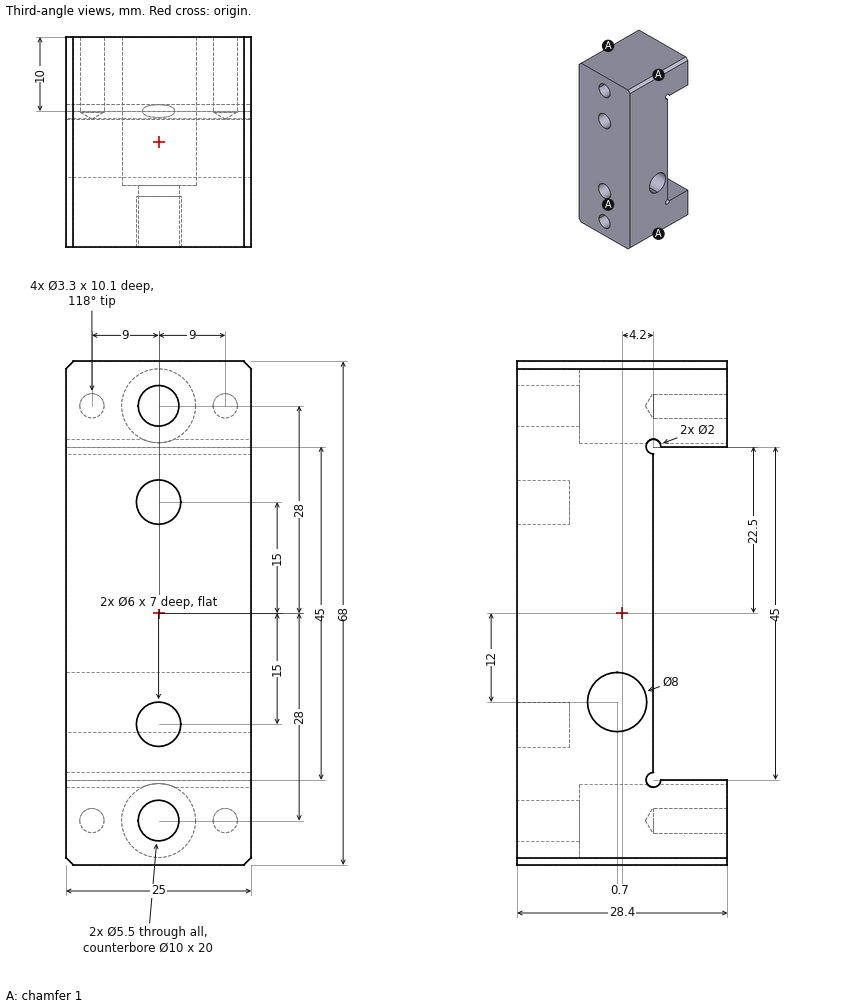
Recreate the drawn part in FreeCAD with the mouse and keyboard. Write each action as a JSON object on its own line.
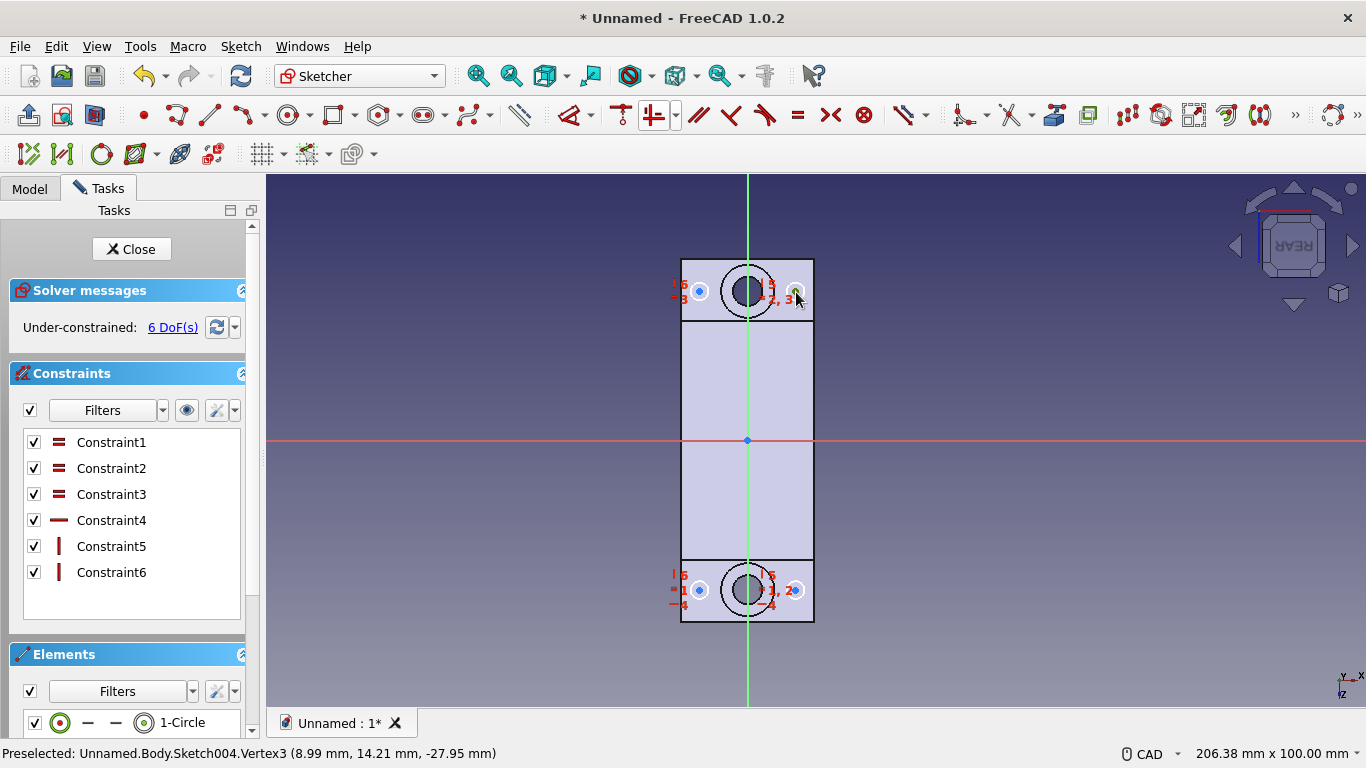
{"action": "left_click", "coordinate": [700, 292]}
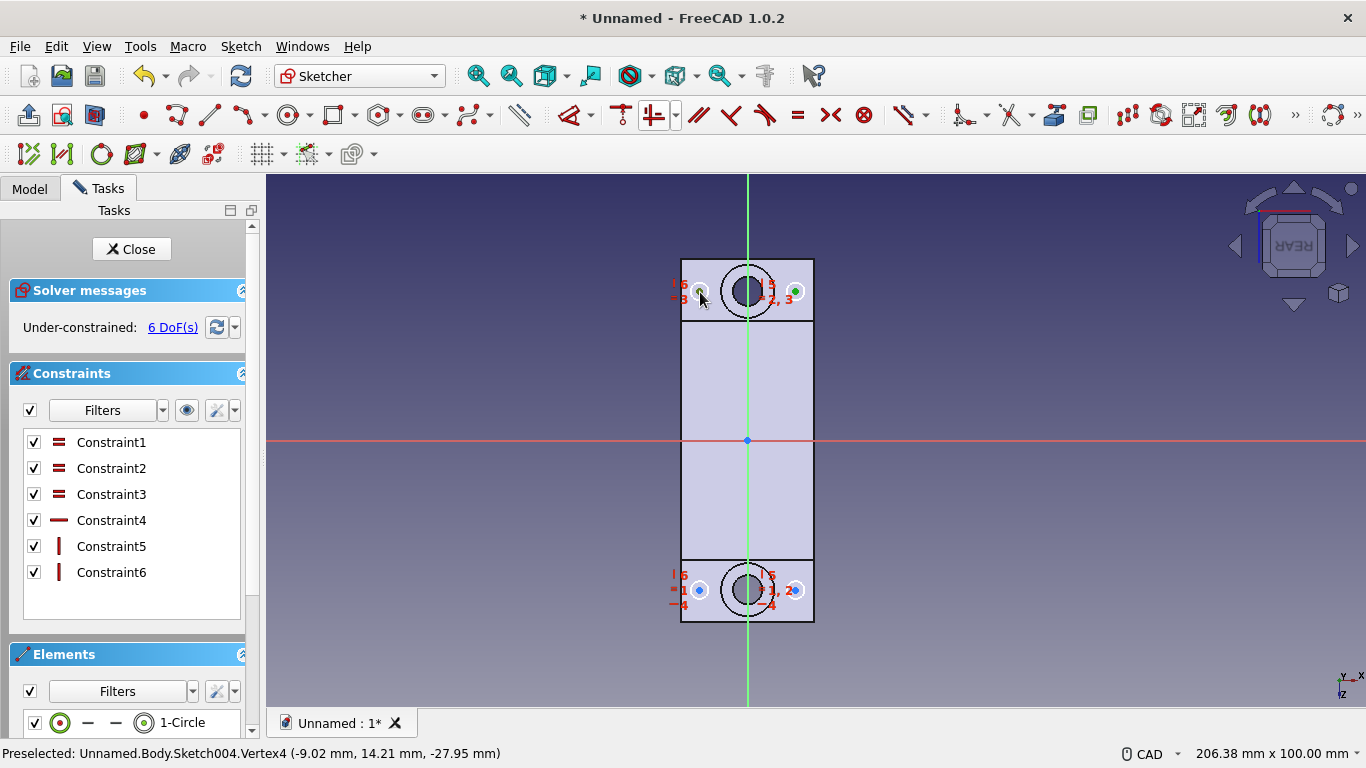
{"action": "key", "text": "h"}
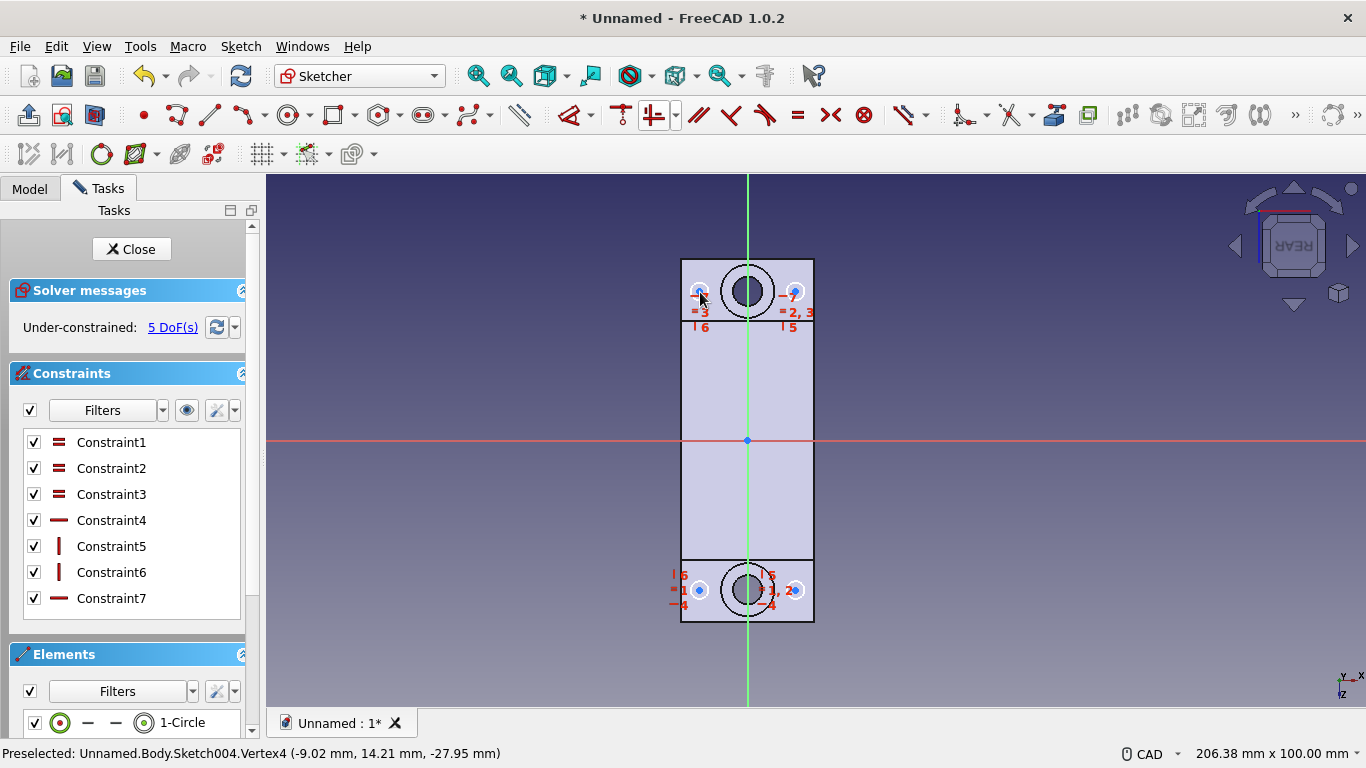
{"action": "left_click", "coordinate": [568, 116]}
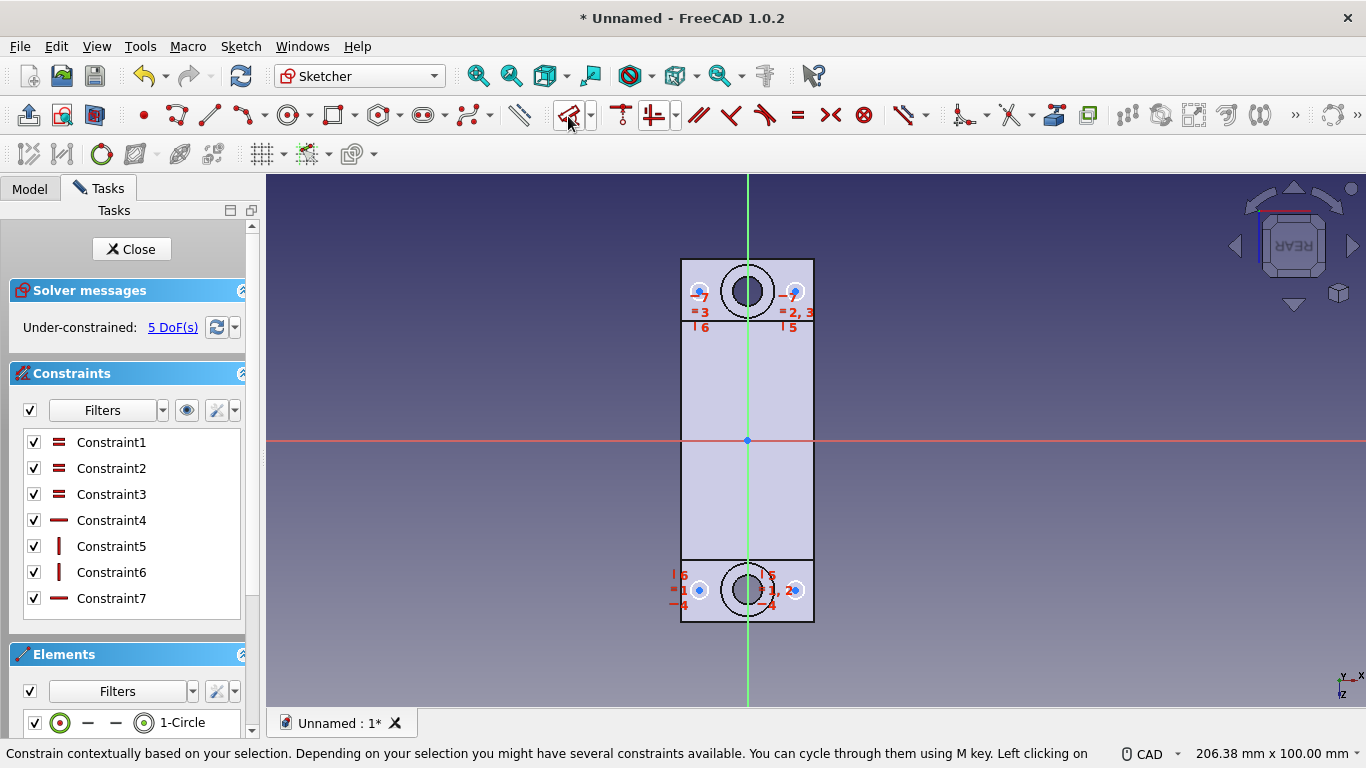
{"action": "scroll", "coordinate": [706, 584], "scroll_direction": "up", "scroll_amount": 5}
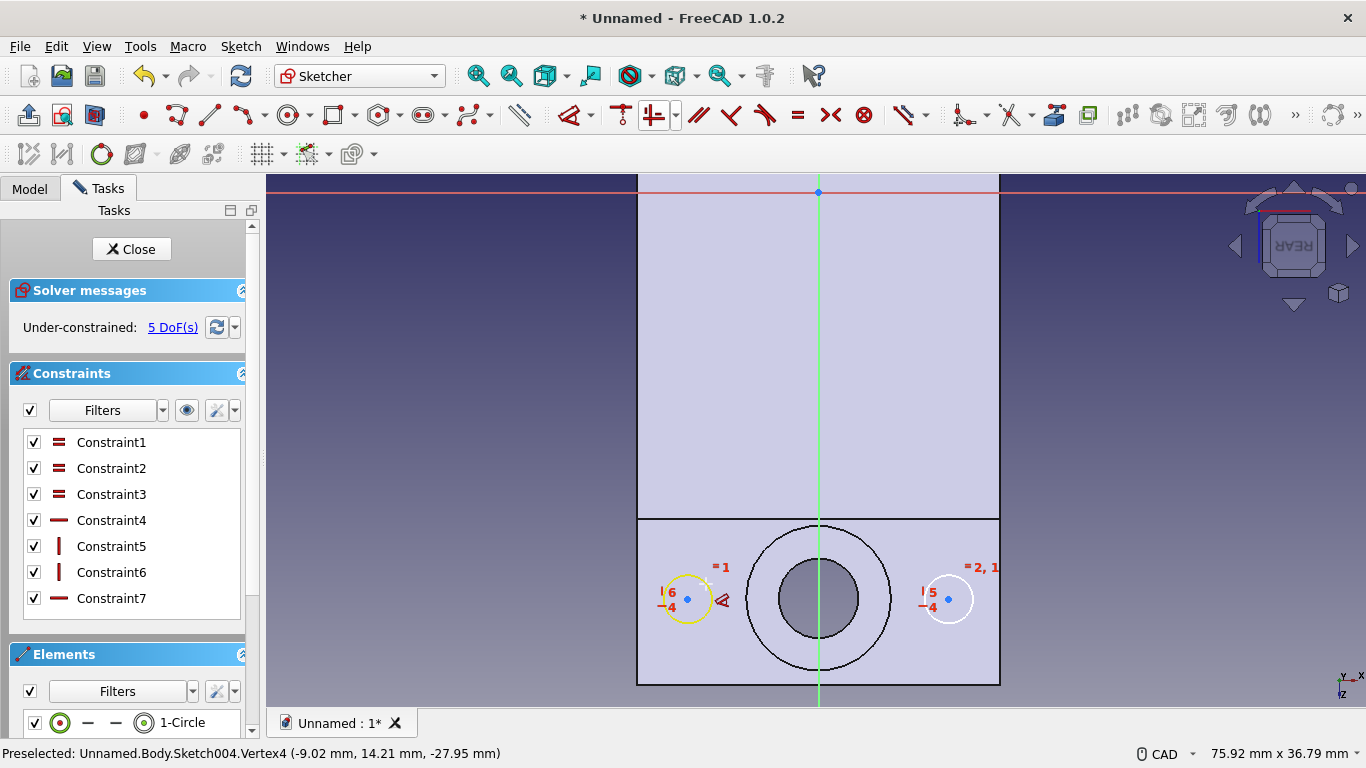
{"action": "left_click", "coordinate": [705, 582]}
{"action": "left_click", "coordinate": [727, 559]}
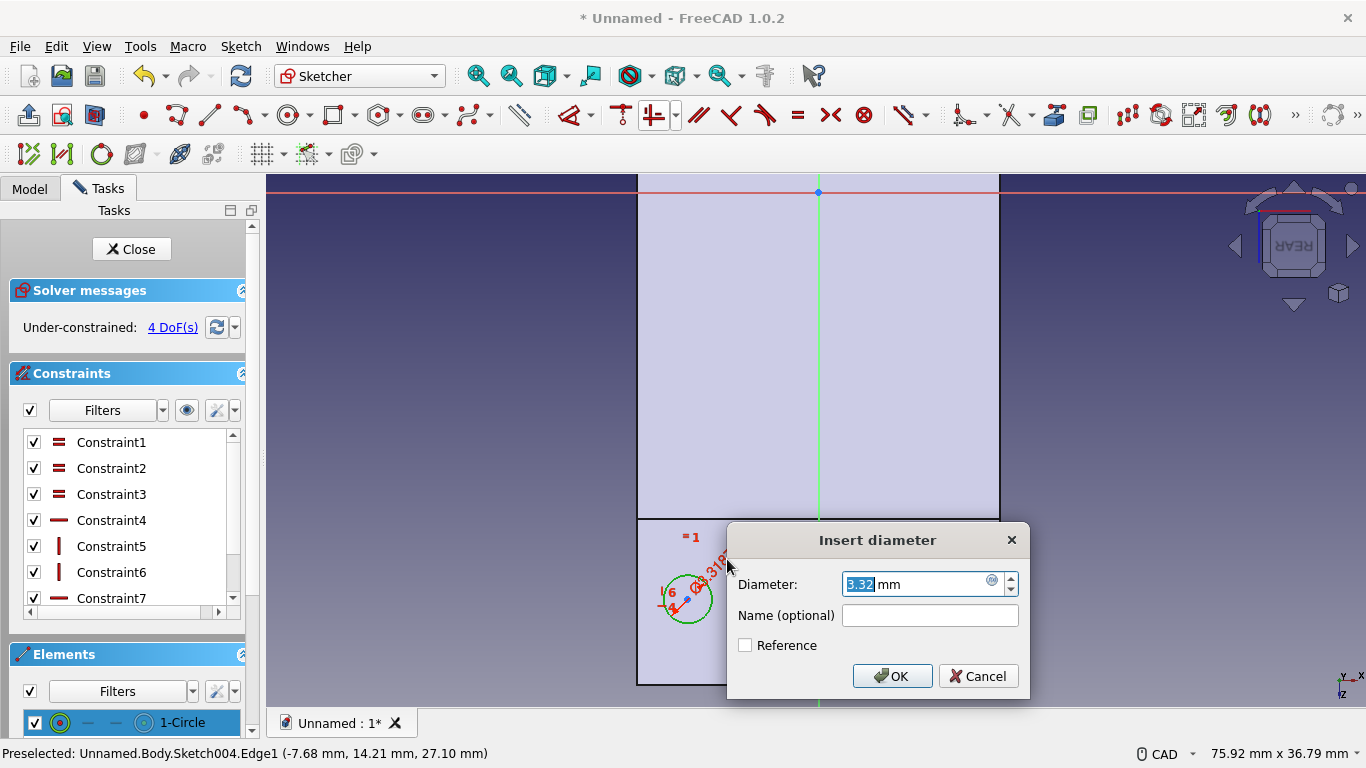
{"action": "type", "text": "3.3"}
{"action": "key", "text": "Return"}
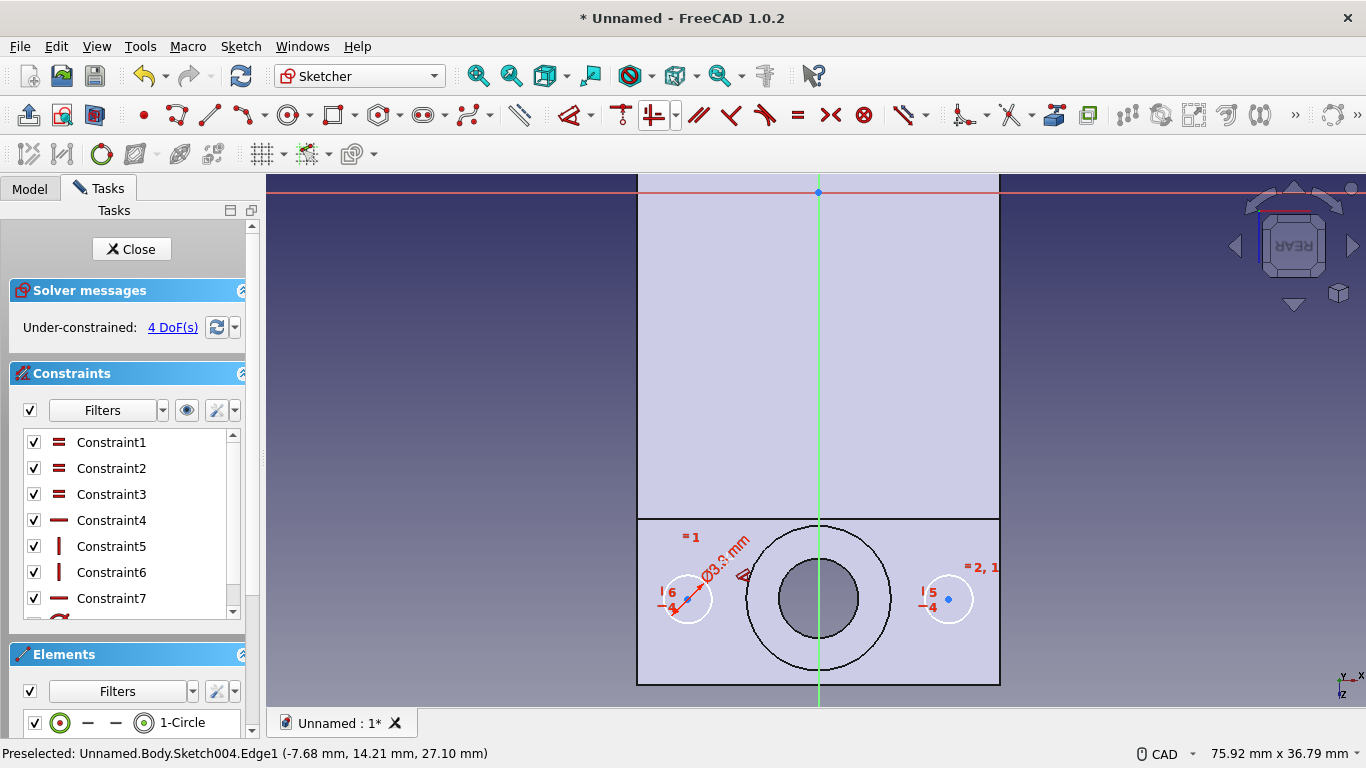
{"action": "left_click", "coordinate": [688, 599]}
{"action": "left_click", "coordinate": [753, 633]}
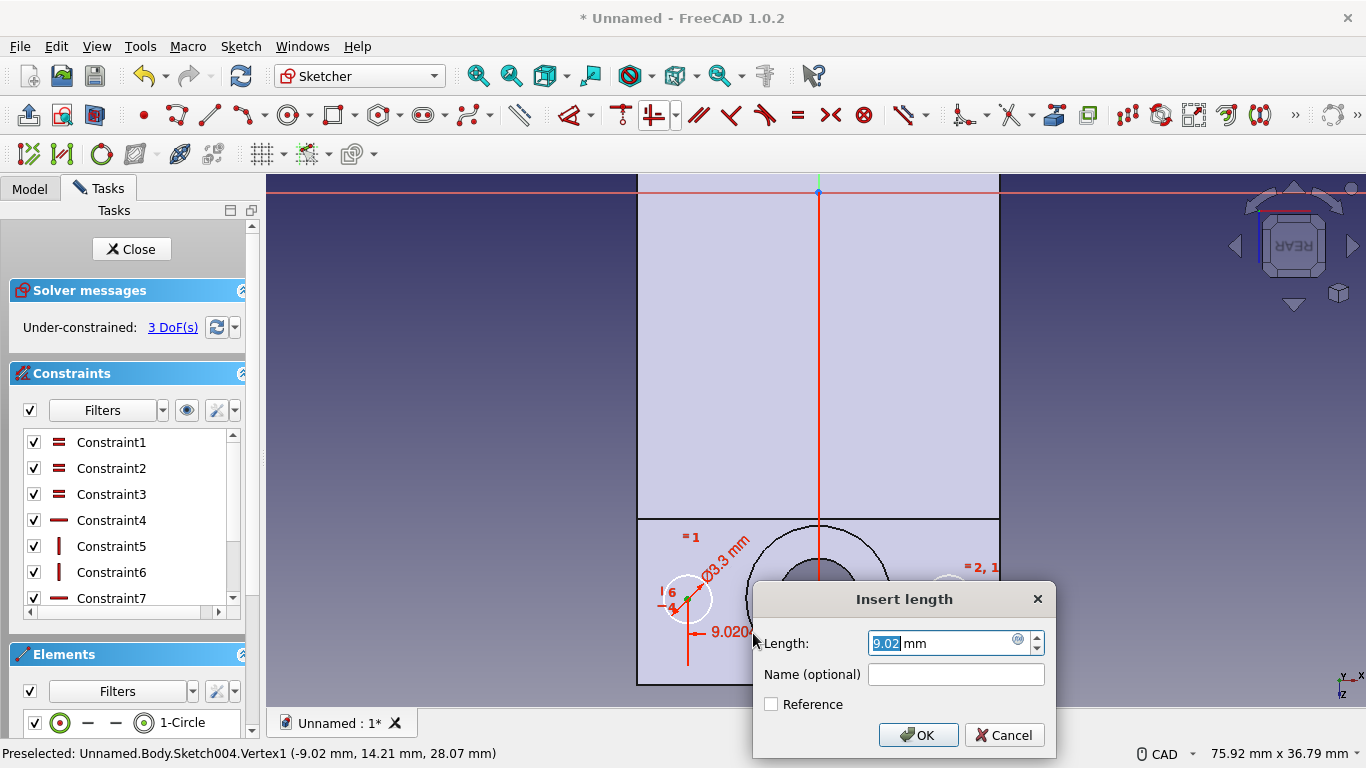
{"action": "type", "text": "9"}
{"action": "key", "text": "Return"}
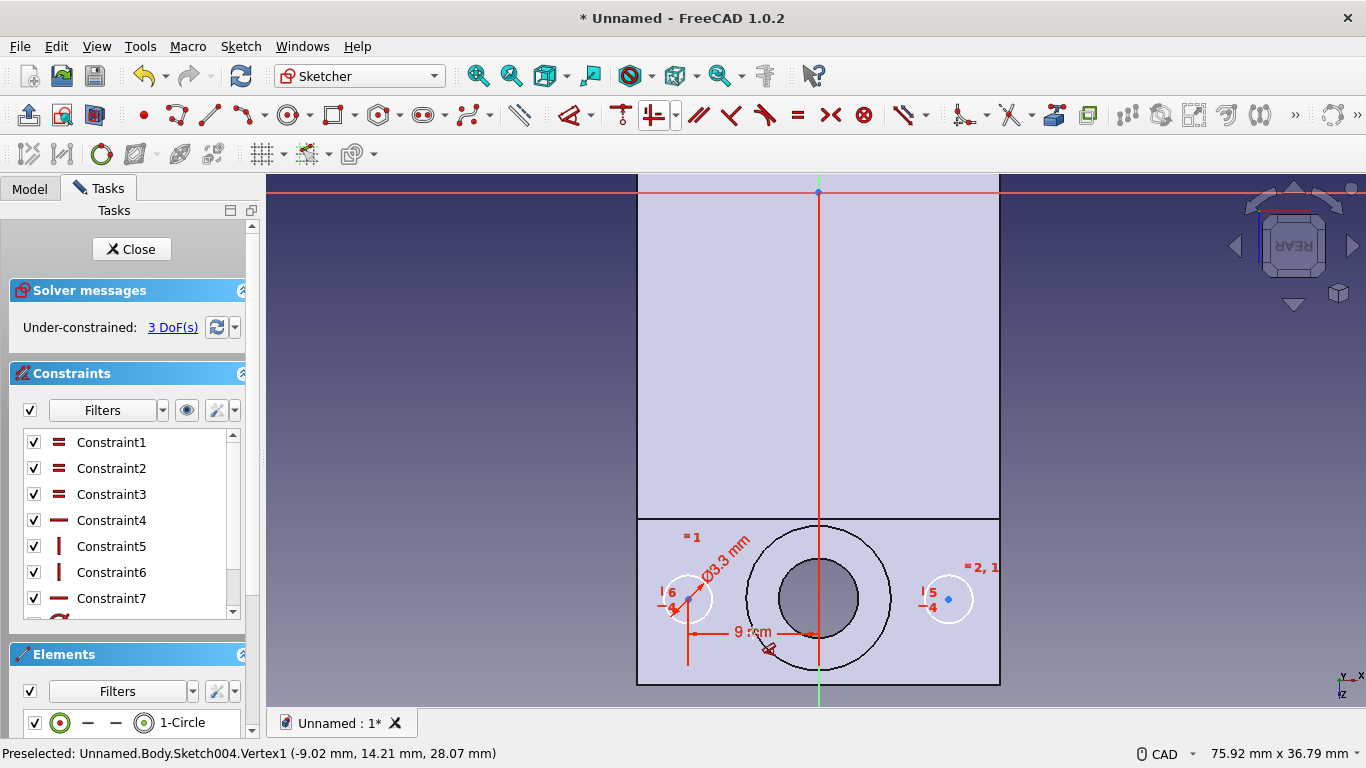
{"action": "left_click", "coordinate": [949, 599]}
{"action": "left_click", "coordinate": [884, 633]}